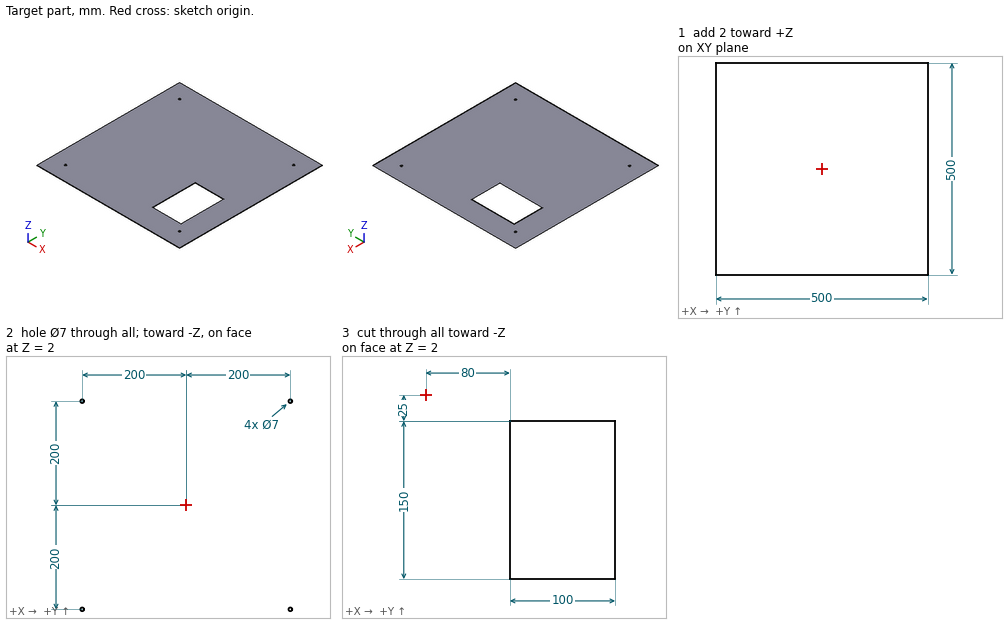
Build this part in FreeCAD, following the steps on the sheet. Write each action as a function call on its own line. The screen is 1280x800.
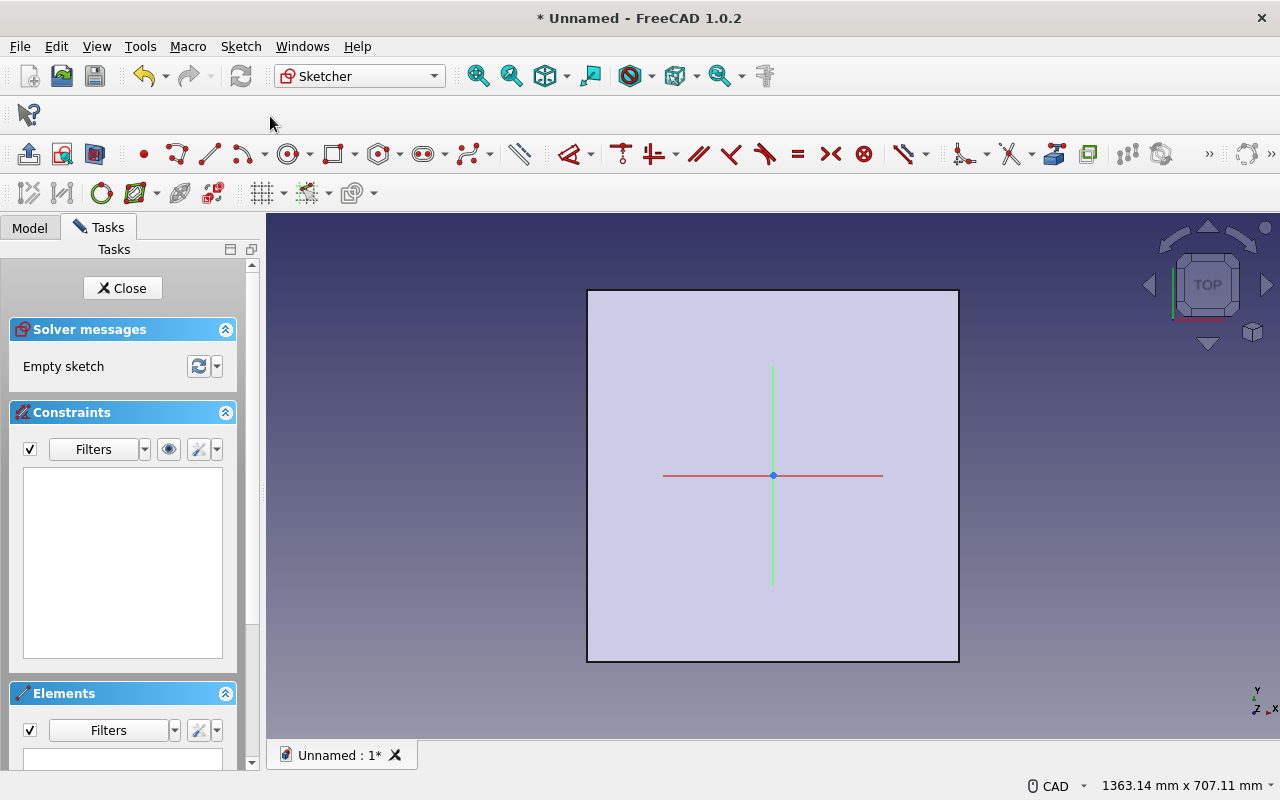
key(g)
key(c)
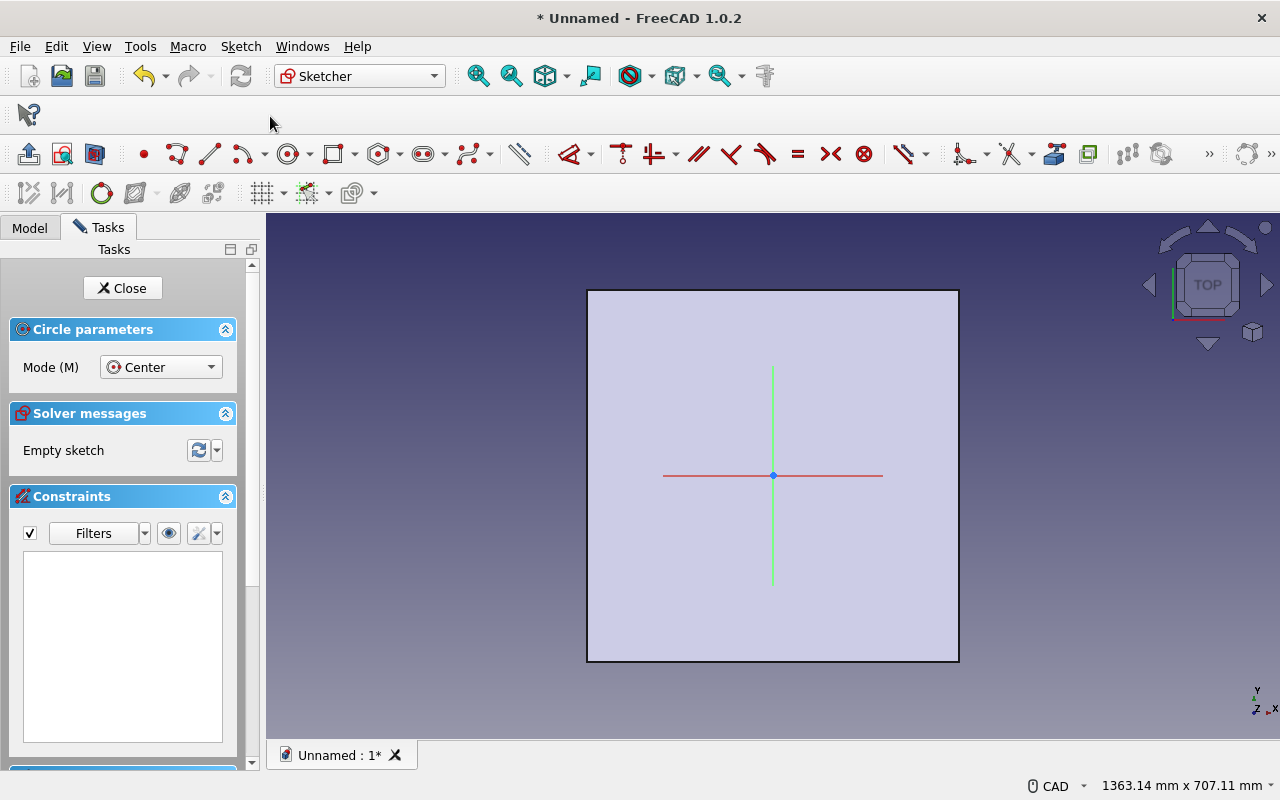
scroll(624, 327, up, 11)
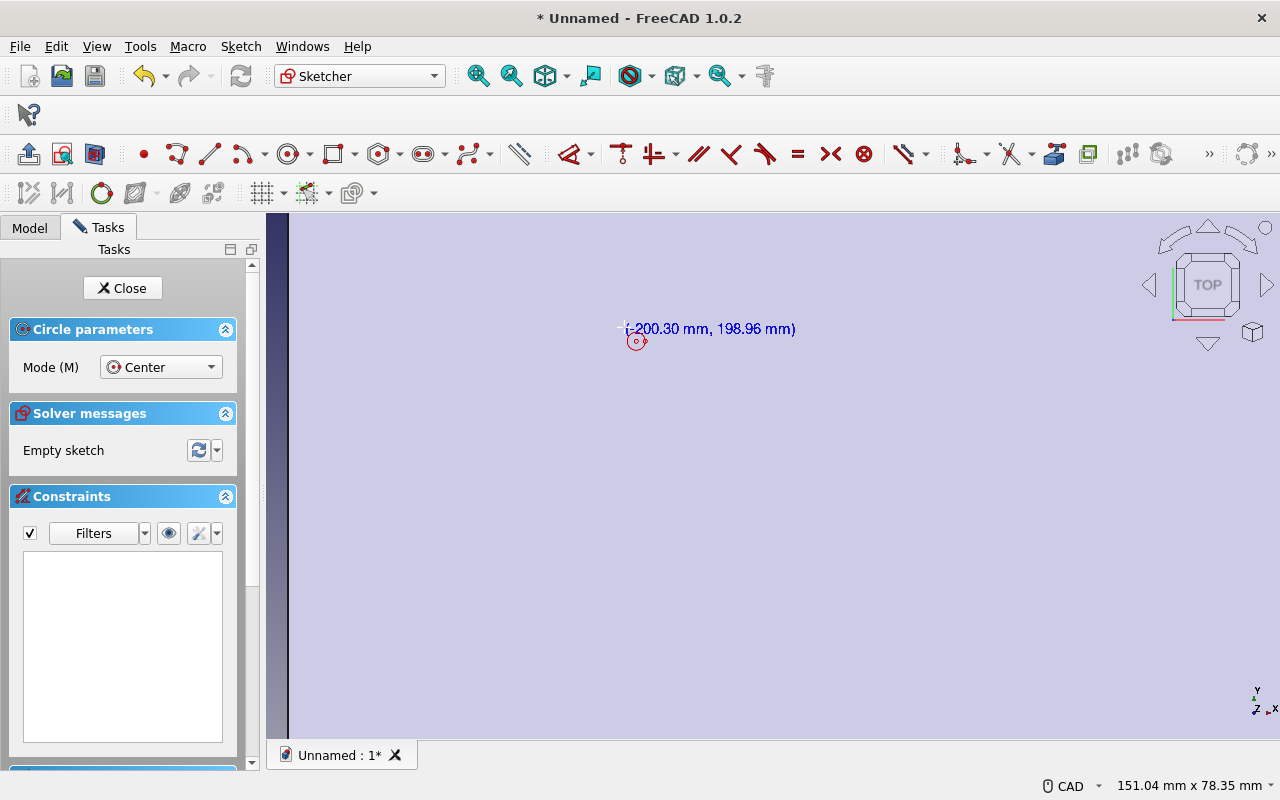
scroll(547, 327, down, 11)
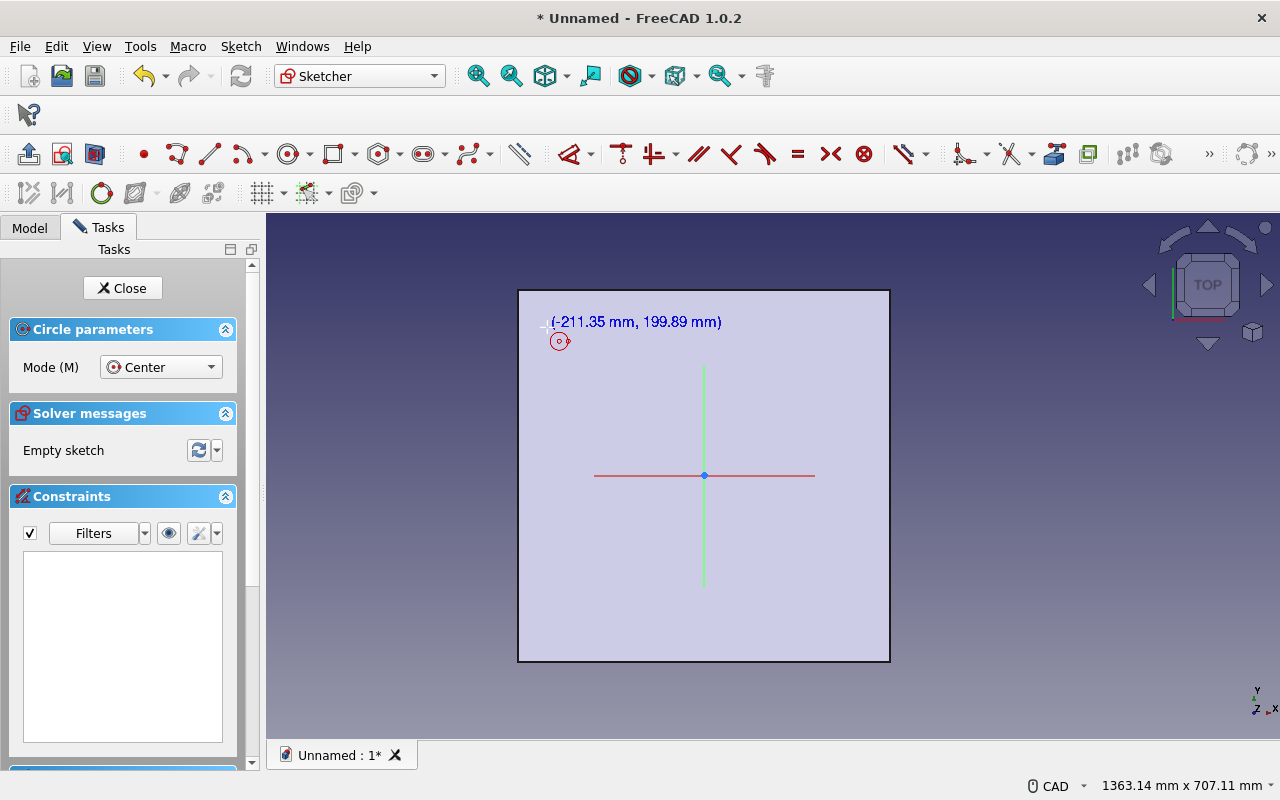
click(556, 327)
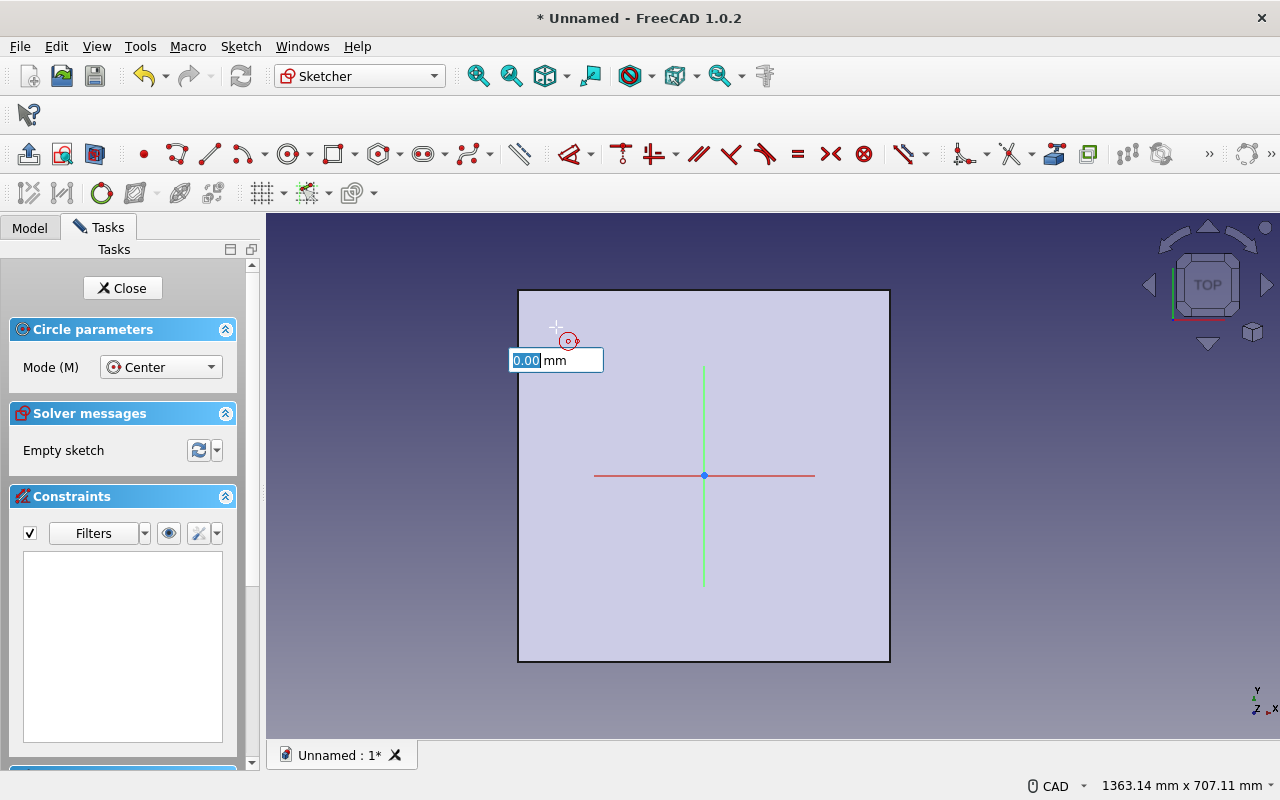
scroll(558, 325, up, 10)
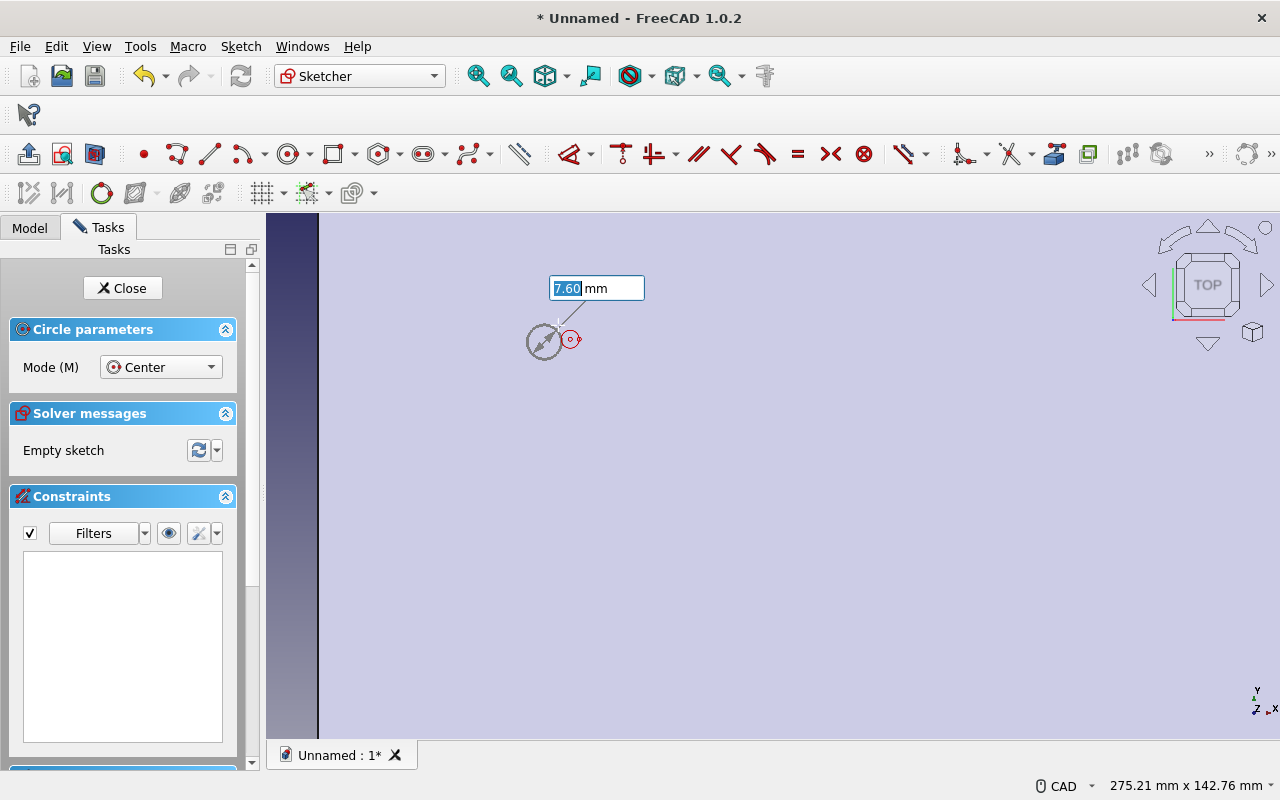
click(553, 326)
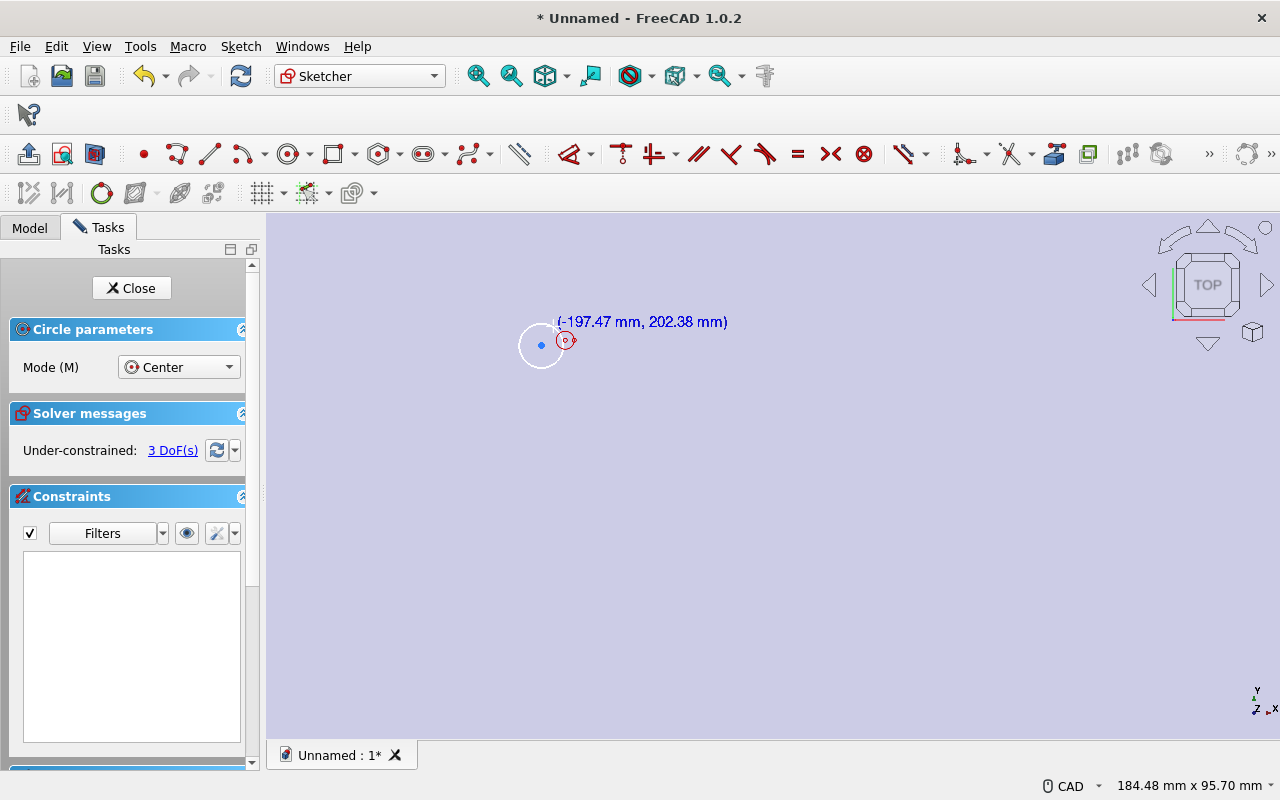
scroll(558, 325, down, 10)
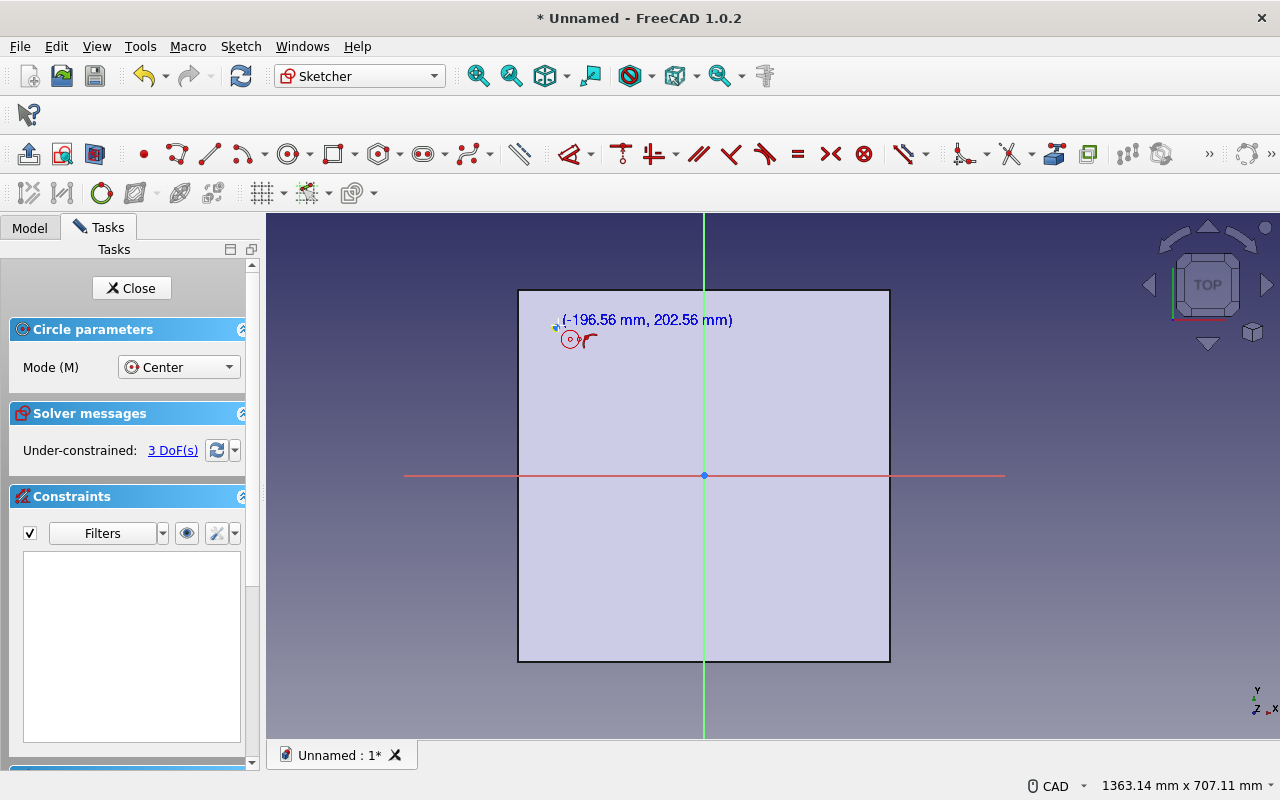
scroll(853, 327, up, 11)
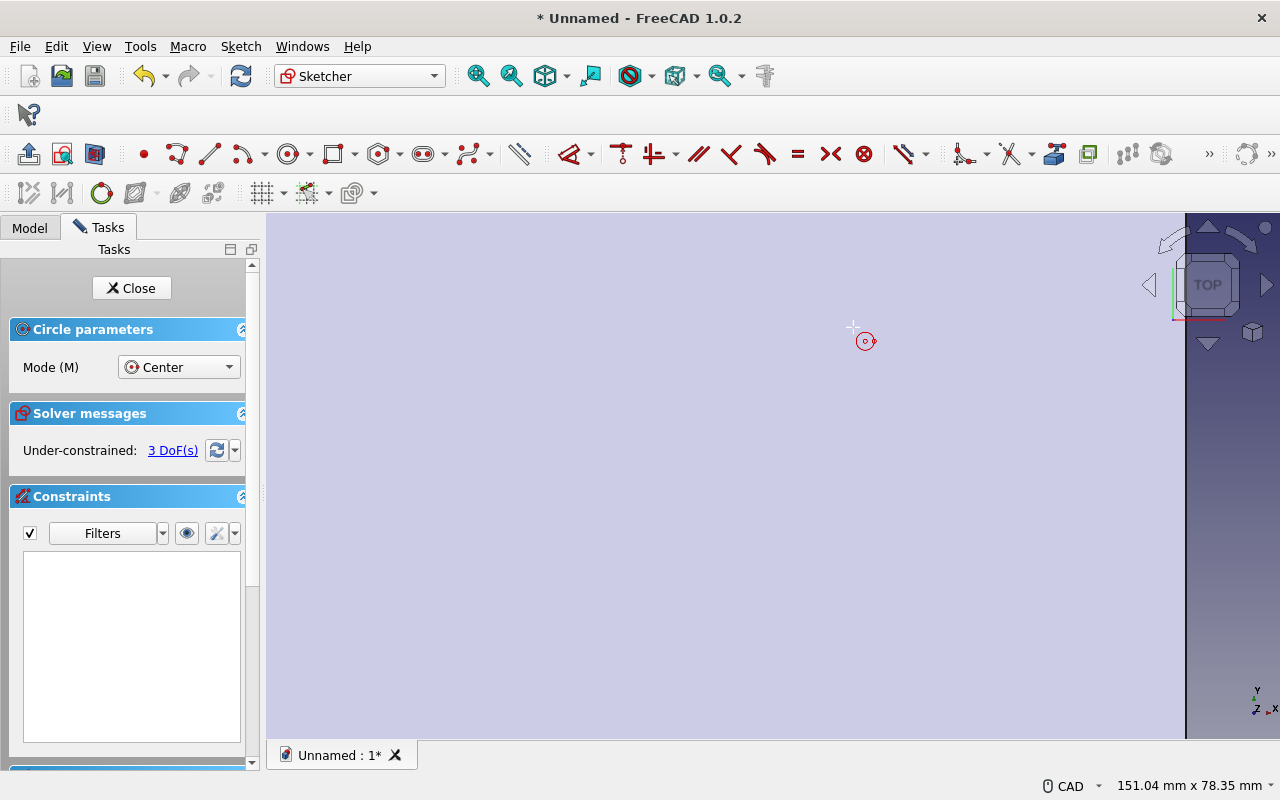
scroll(854, 327, down, 11)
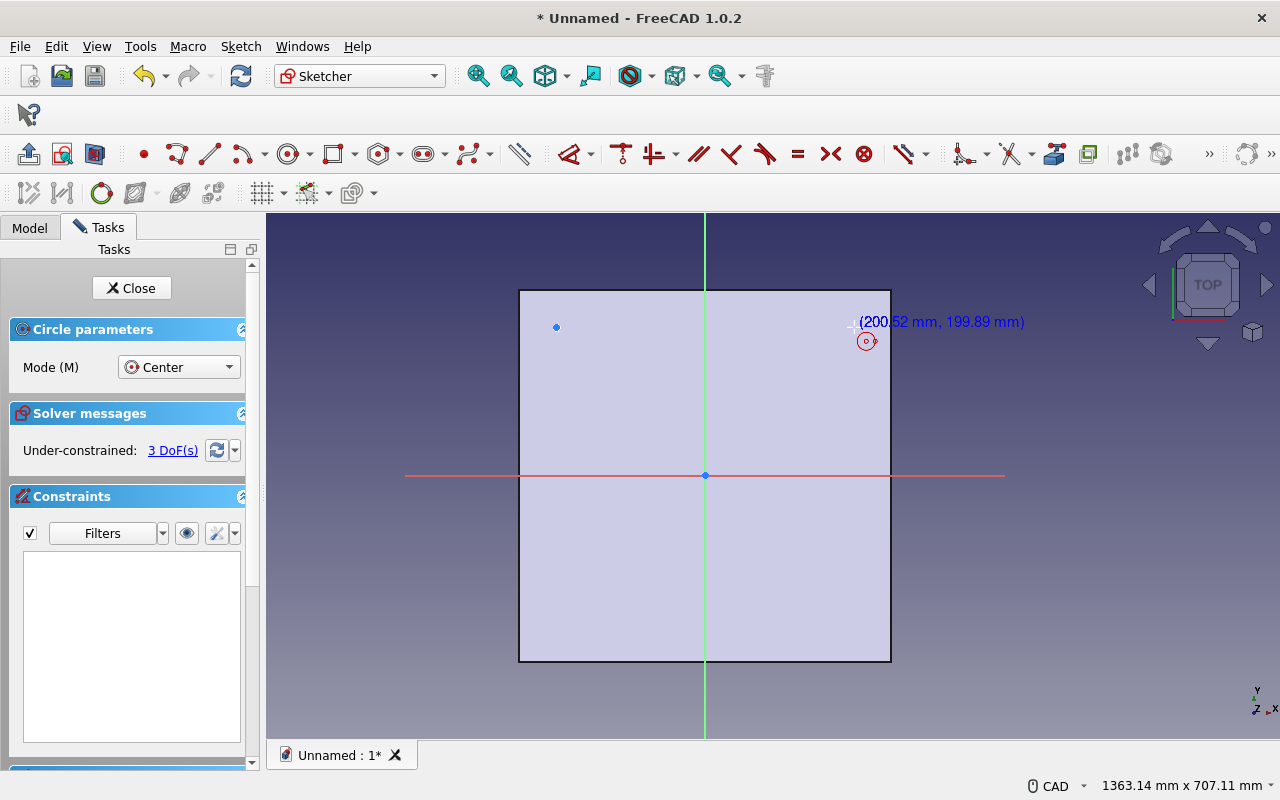
click(854, 327)